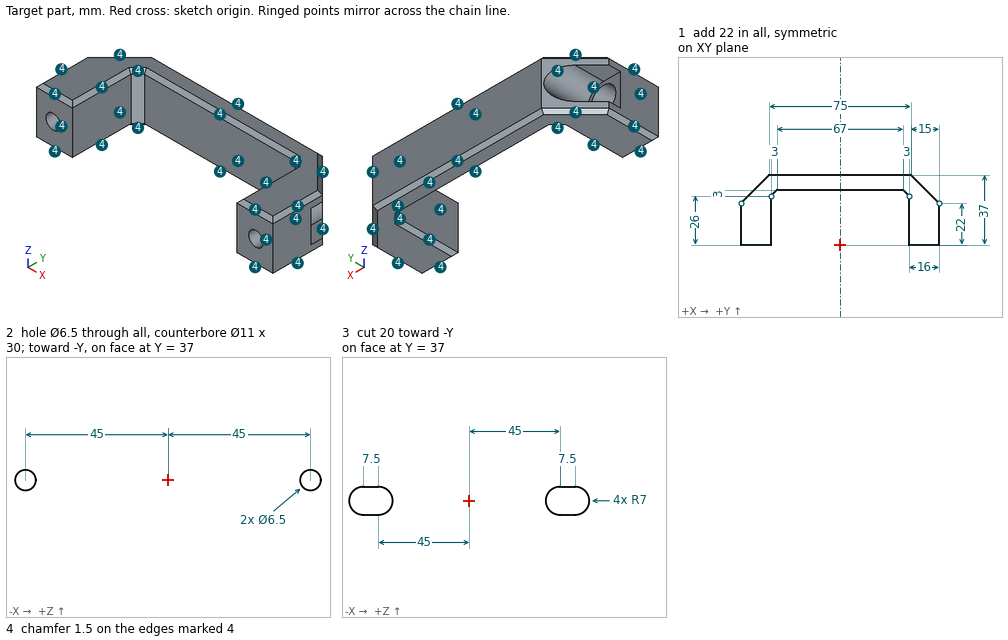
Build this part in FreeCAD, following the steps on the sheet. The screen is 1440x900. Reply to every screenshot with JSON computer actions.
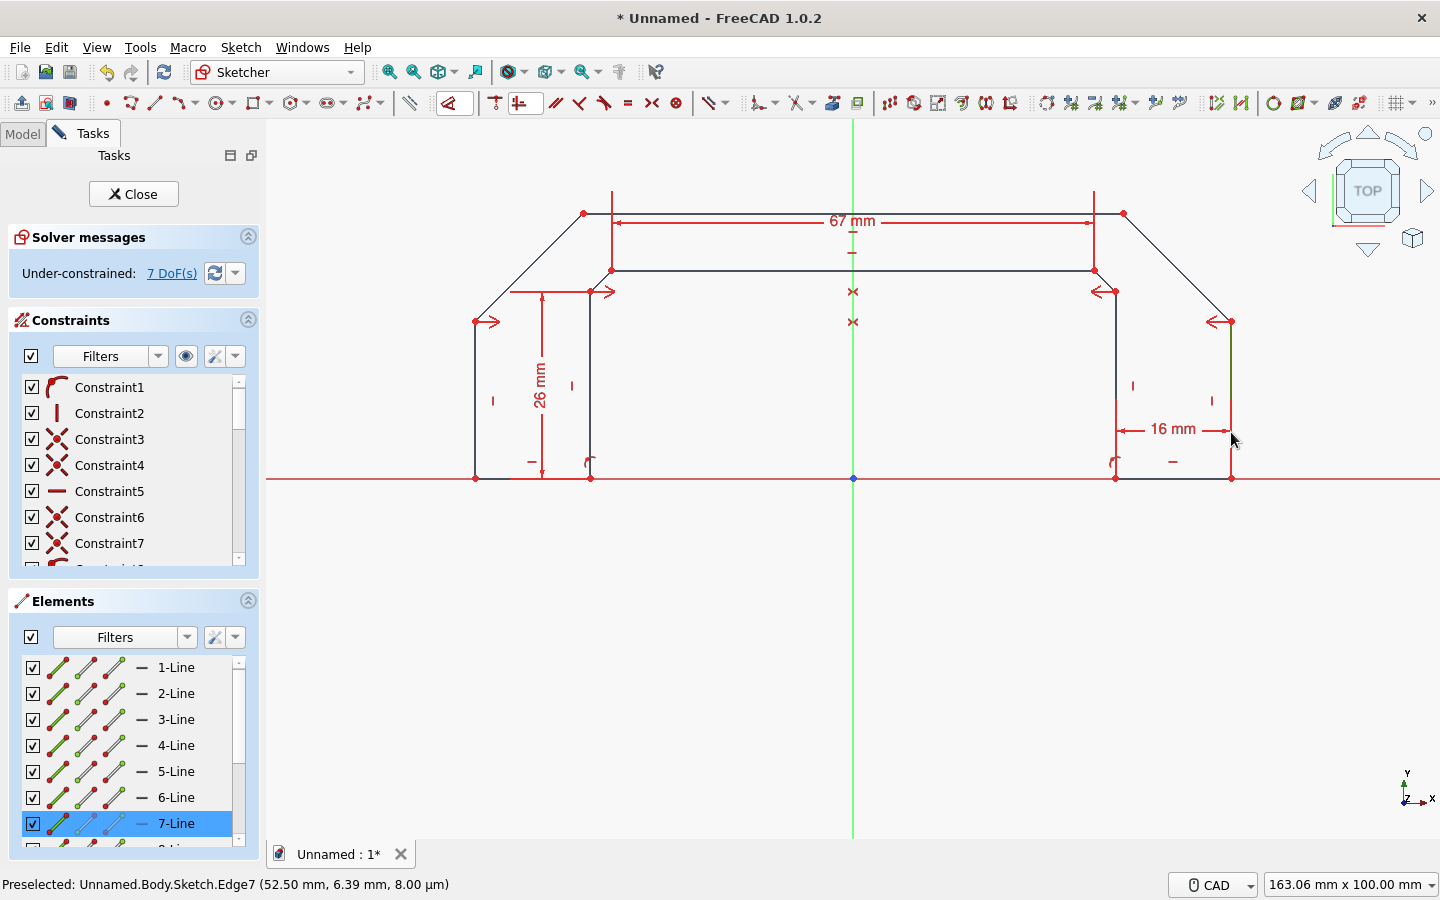
{"action": "left_click", "coordinate": [468, 104]}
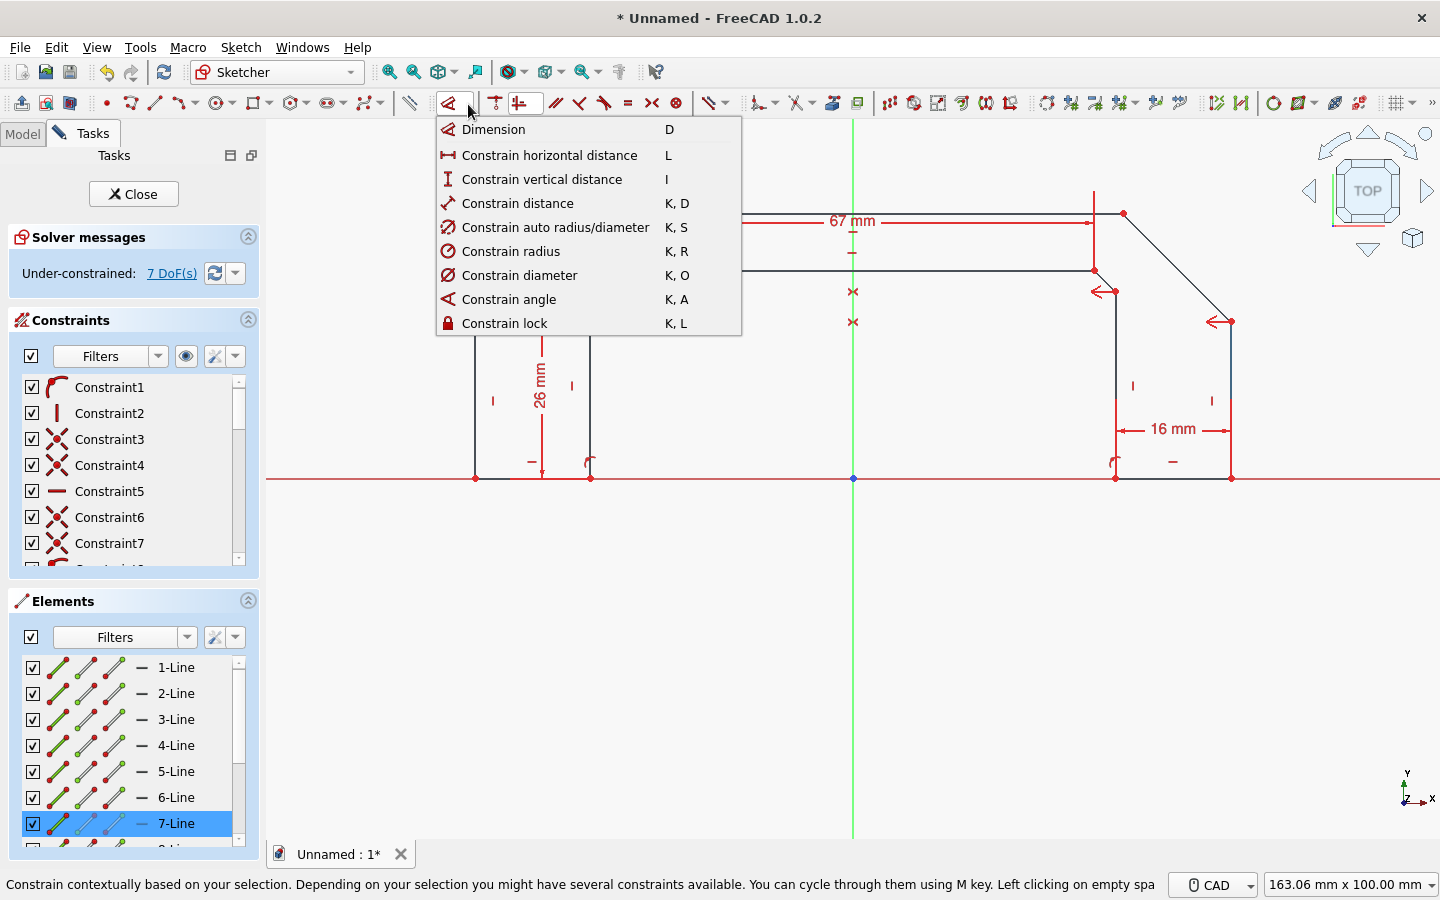
{"action": "left_click", "coordinate": [589, 179]}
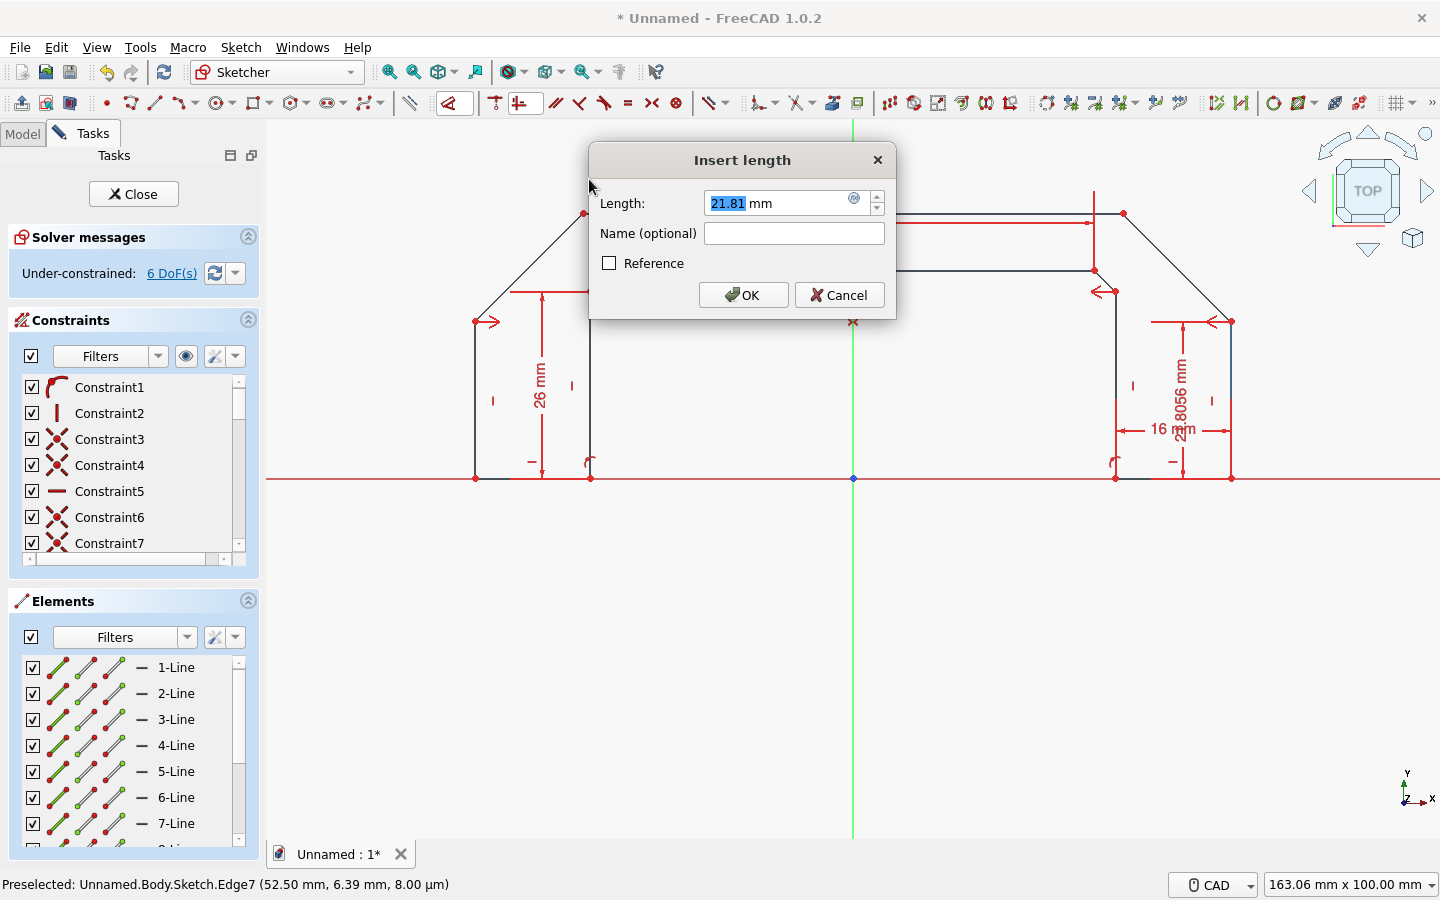
{"action": "type", "text": "22"}
{"action": "key", "text": "Return"}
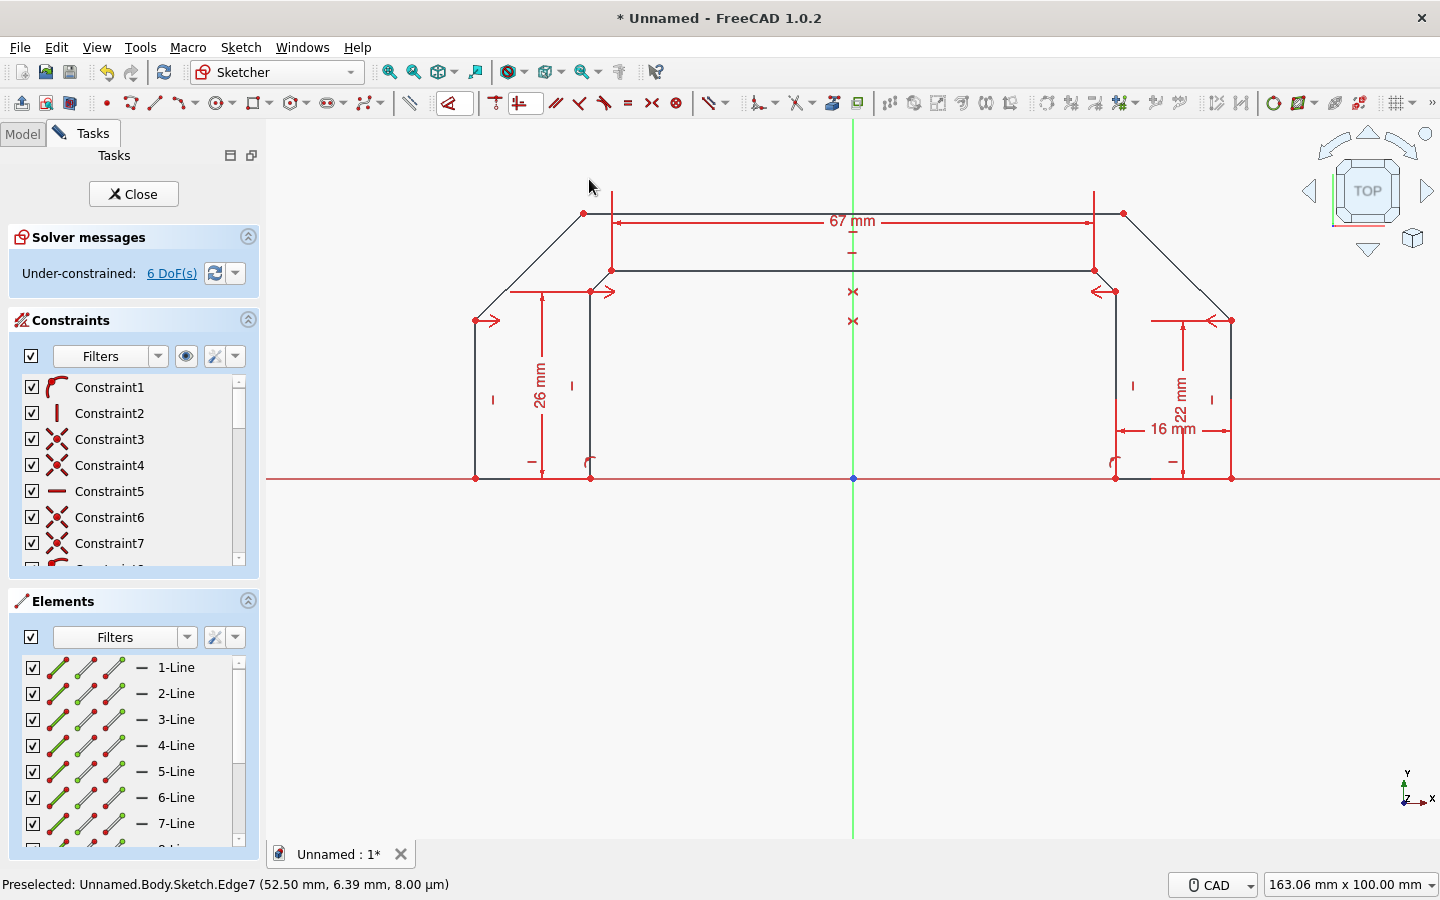
{"action": "left_click", "coordinate": [961, 214]}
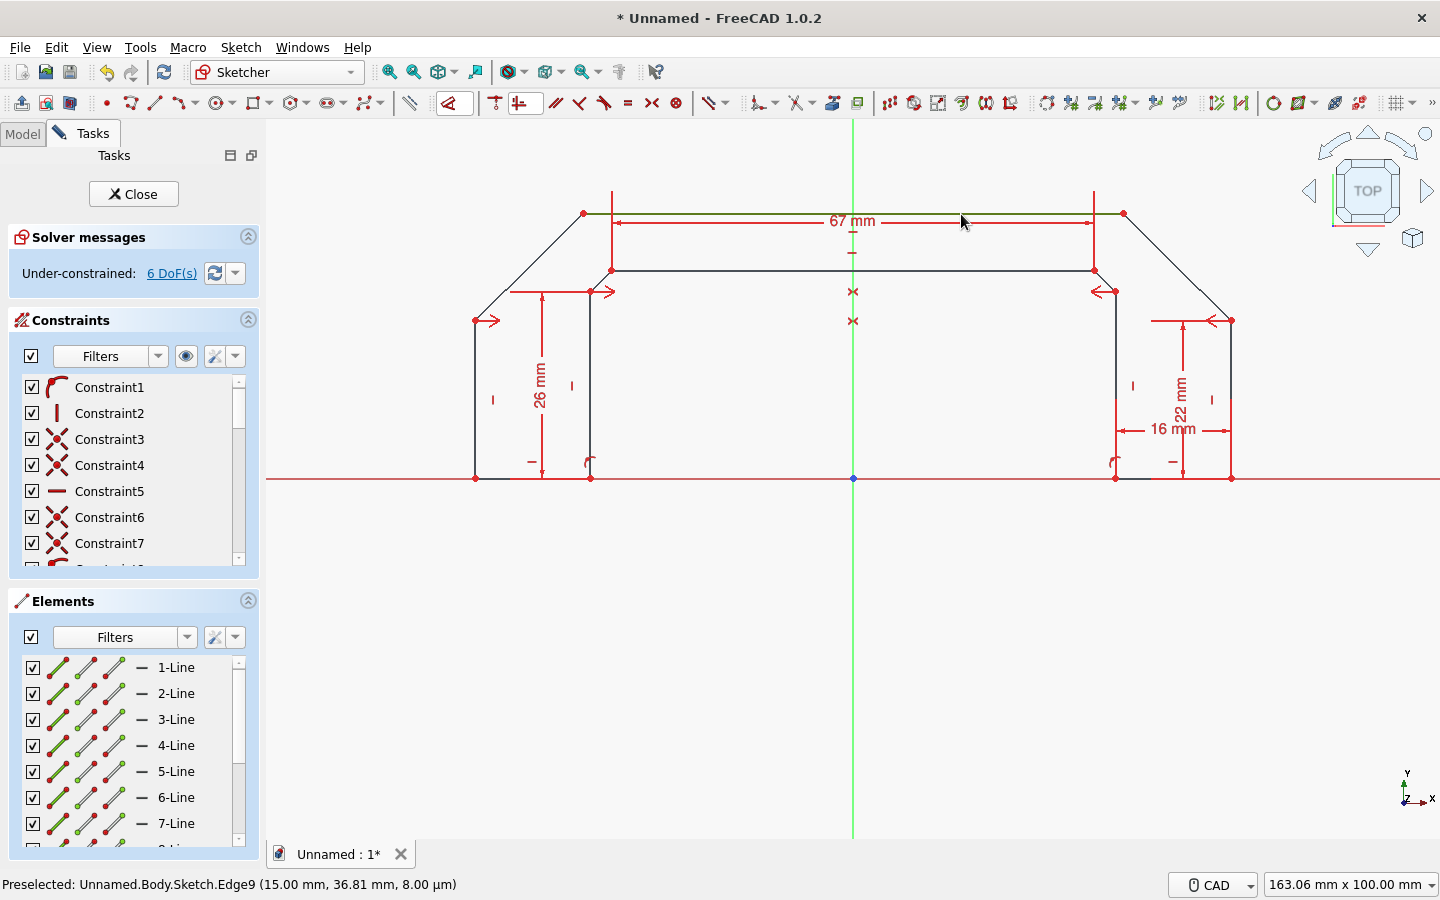
{"action": "left_click", "coordinate": [468, 104]}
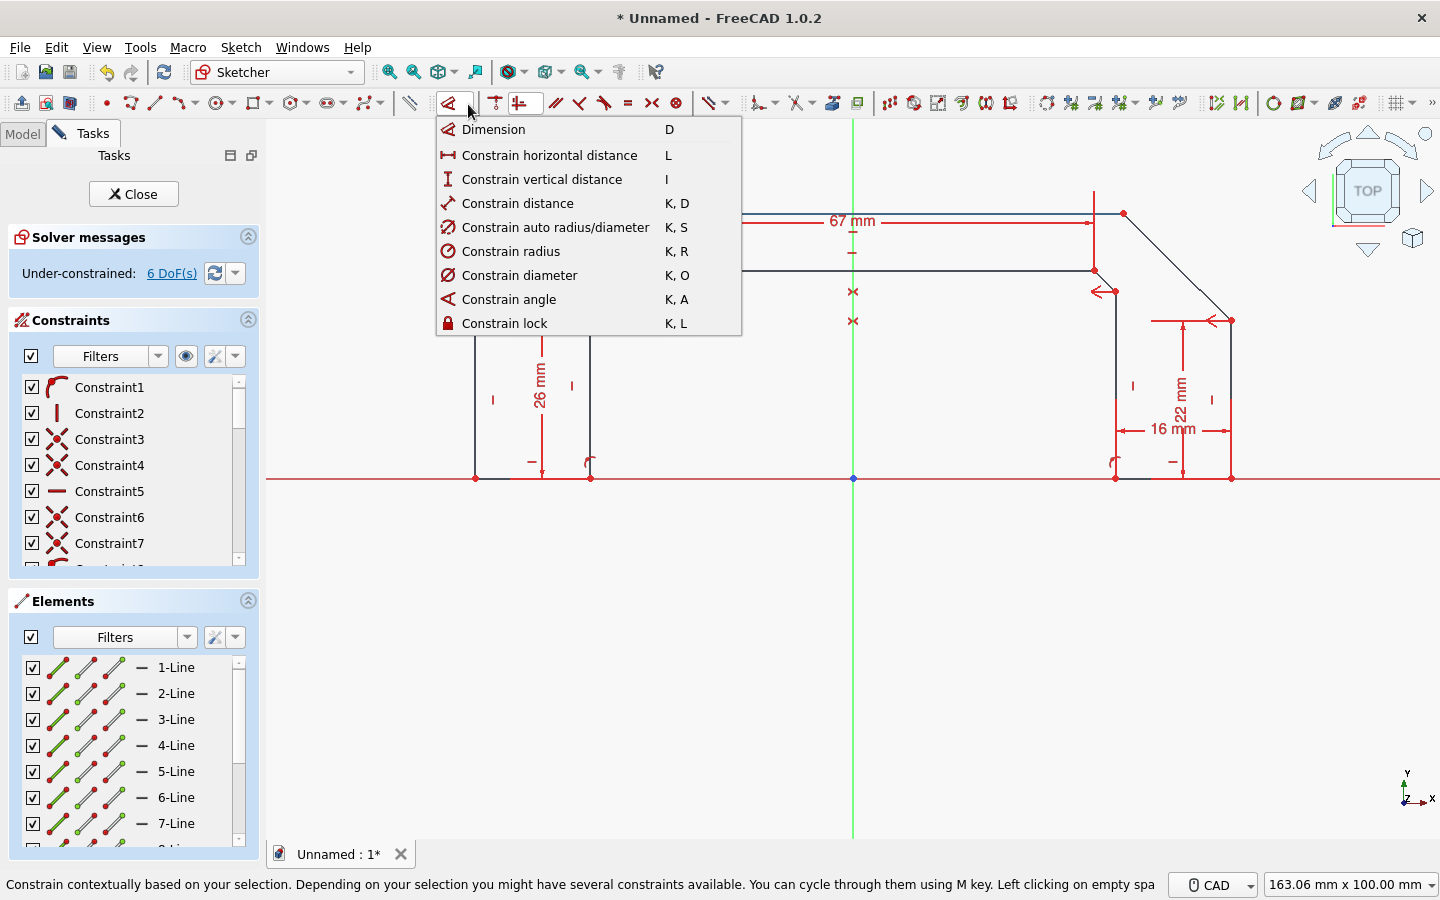
{"action": "left_click", "coordinate": [589, 155]}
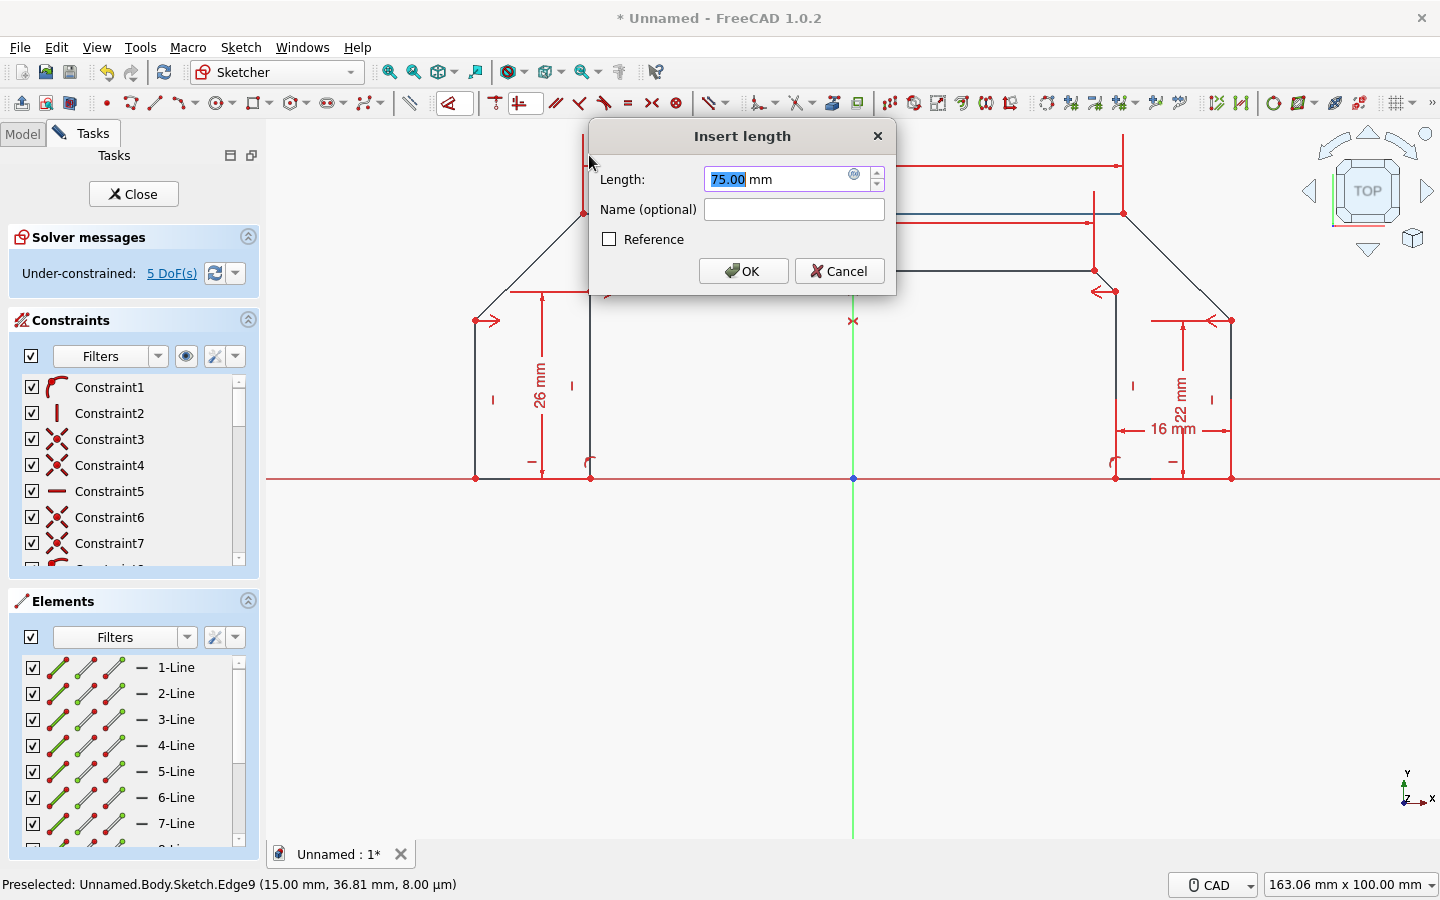
{"action": "type", "text": "75"}
{"action": "key", "text": "Return"}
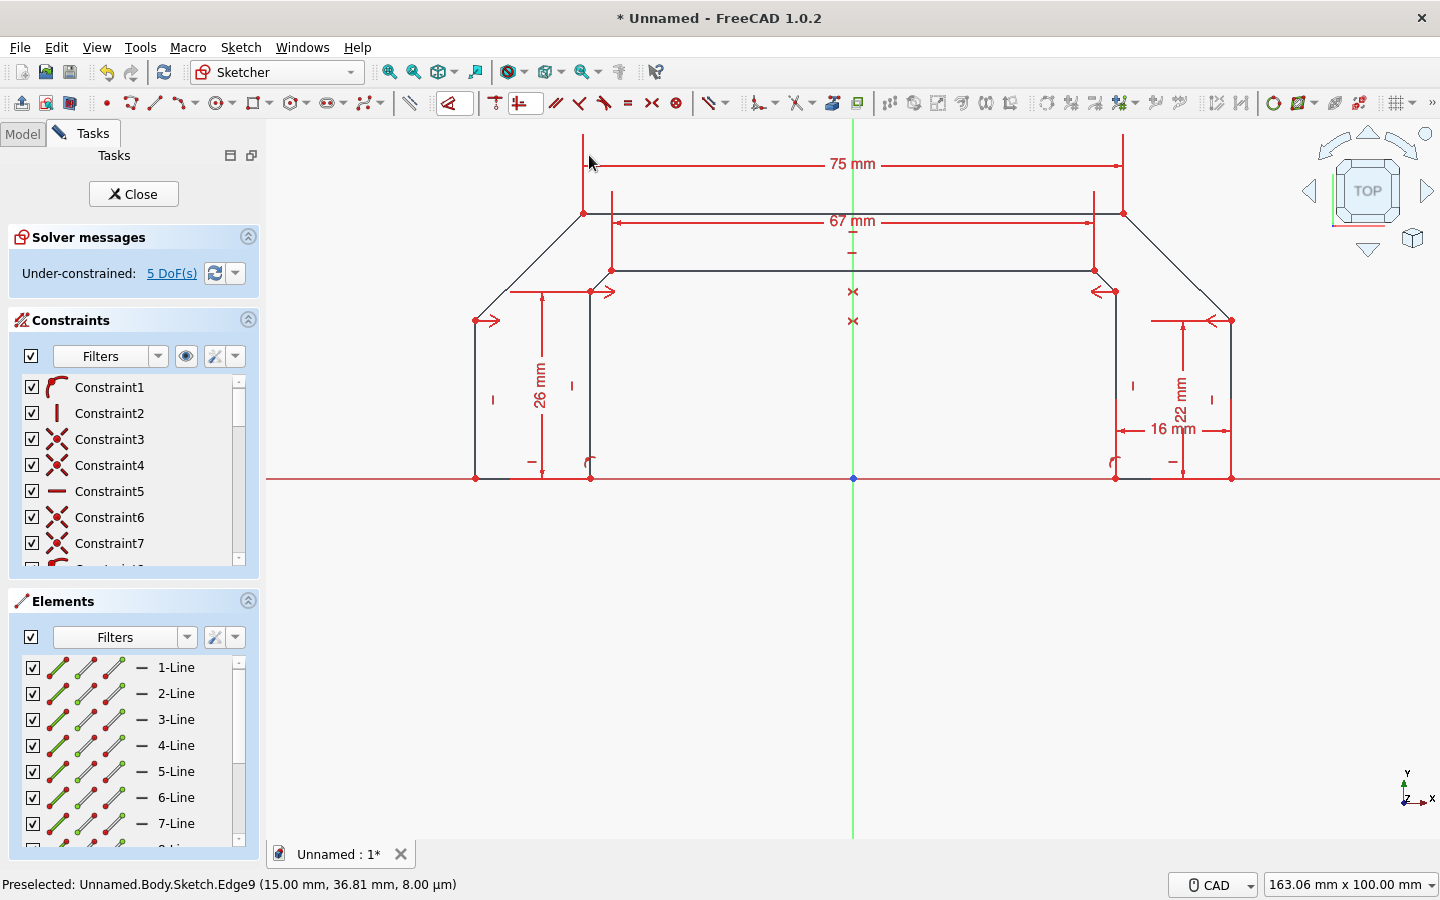
{"action": "scroll", "coordinate": [599, 283], "scroll_direction": "up", "scroll_amount": 4}